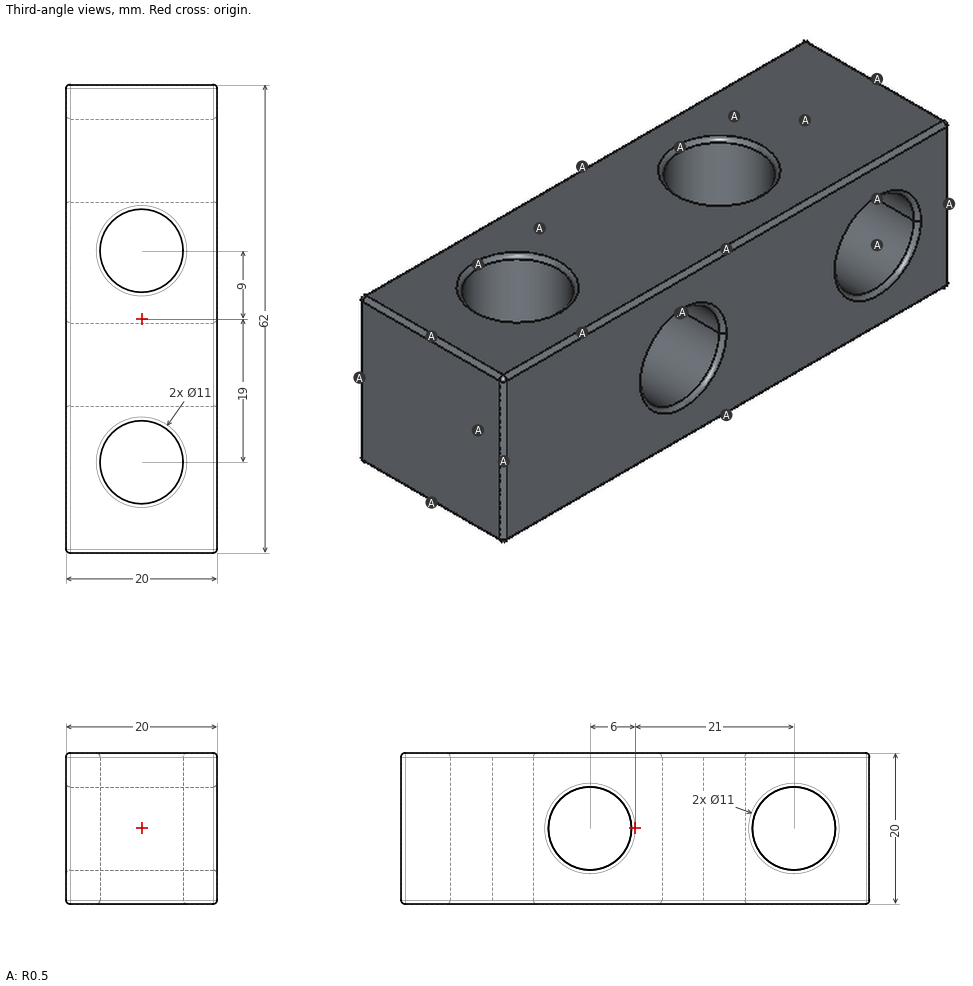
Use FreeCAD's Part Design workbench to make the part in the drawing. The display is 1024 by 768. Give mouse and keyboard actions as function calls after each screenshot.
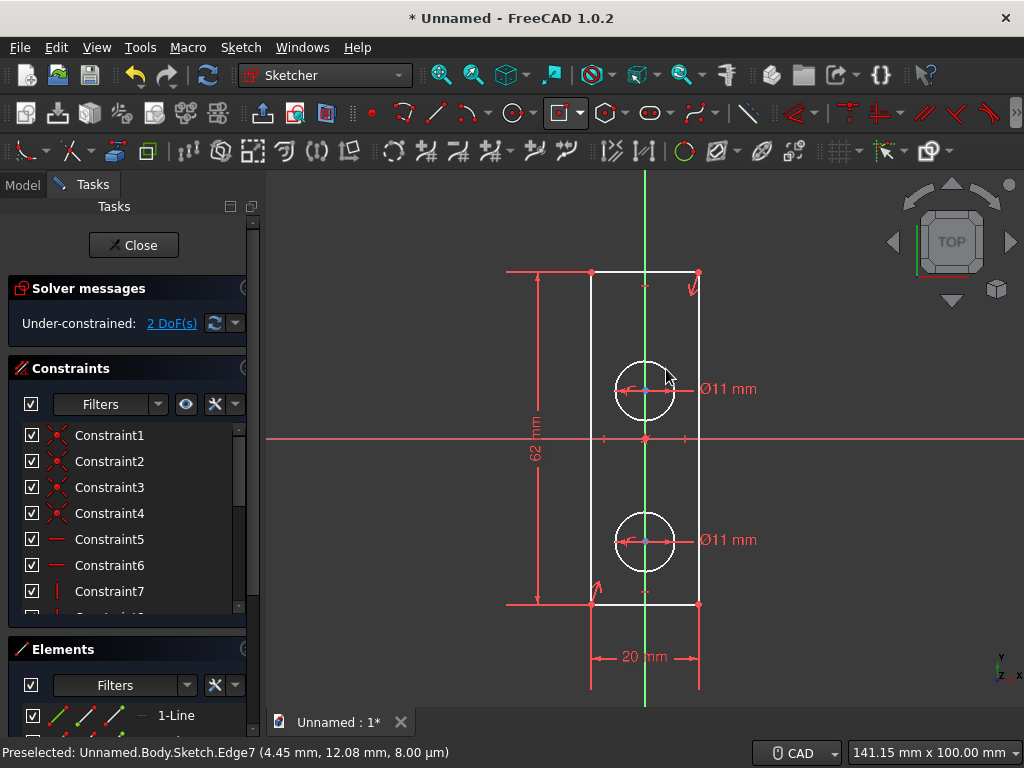
key(d)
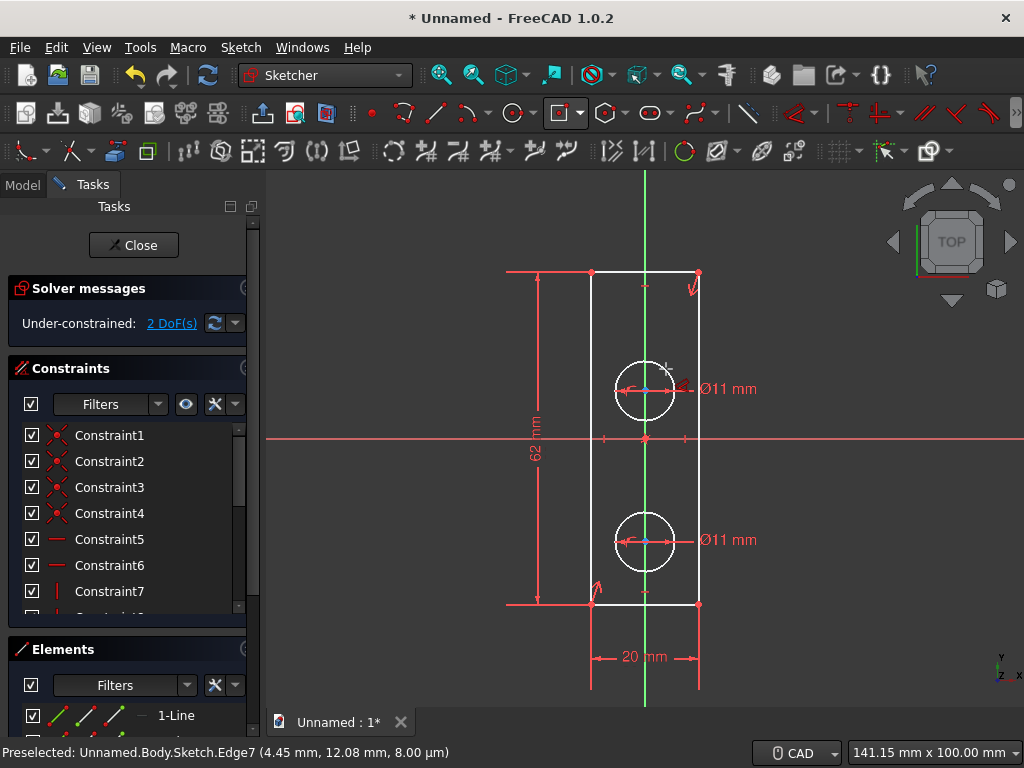
click(645, 391)
click(727, 415)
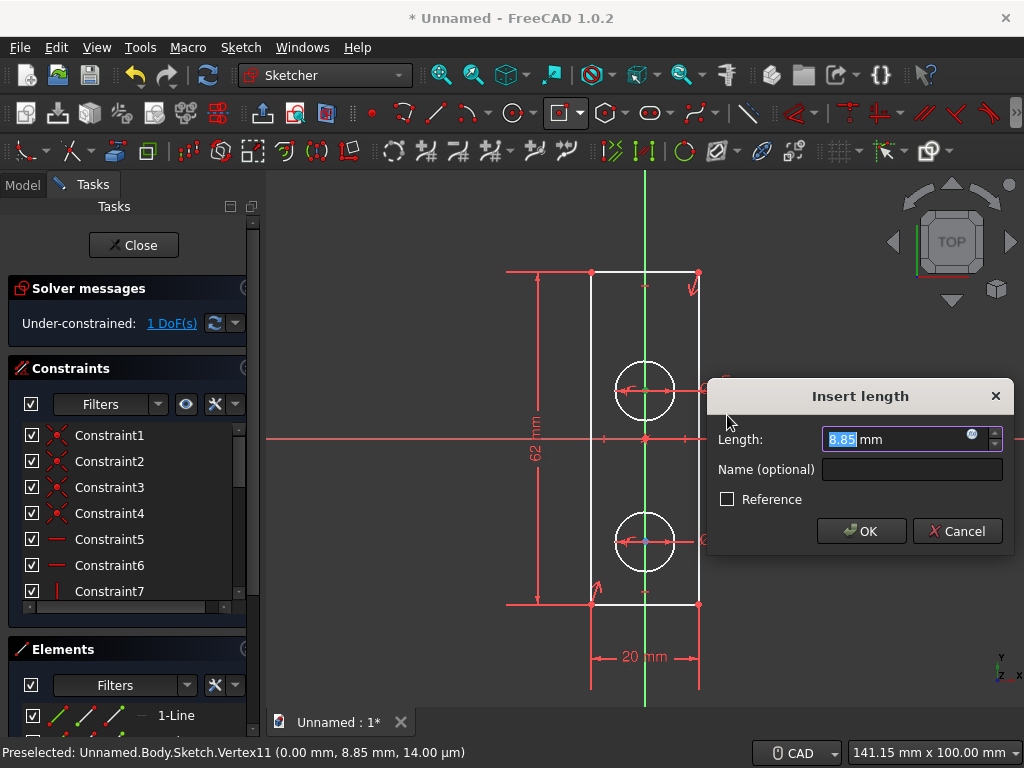
text(9)
key(Return)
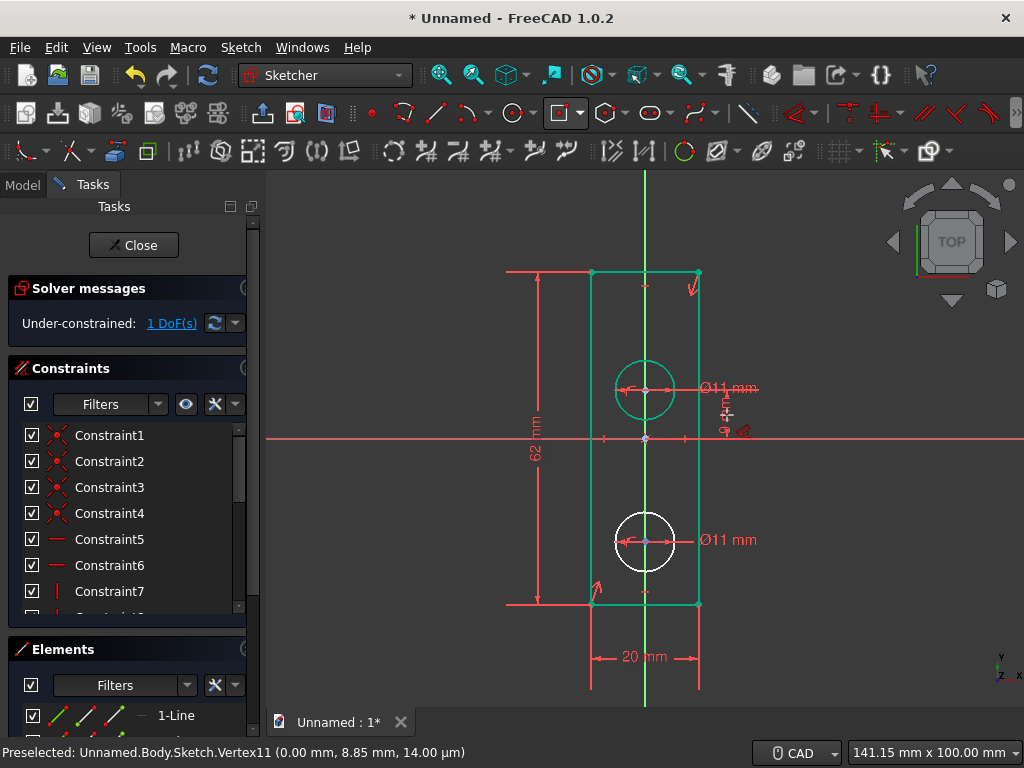
click(645, 542)
click(679, 490)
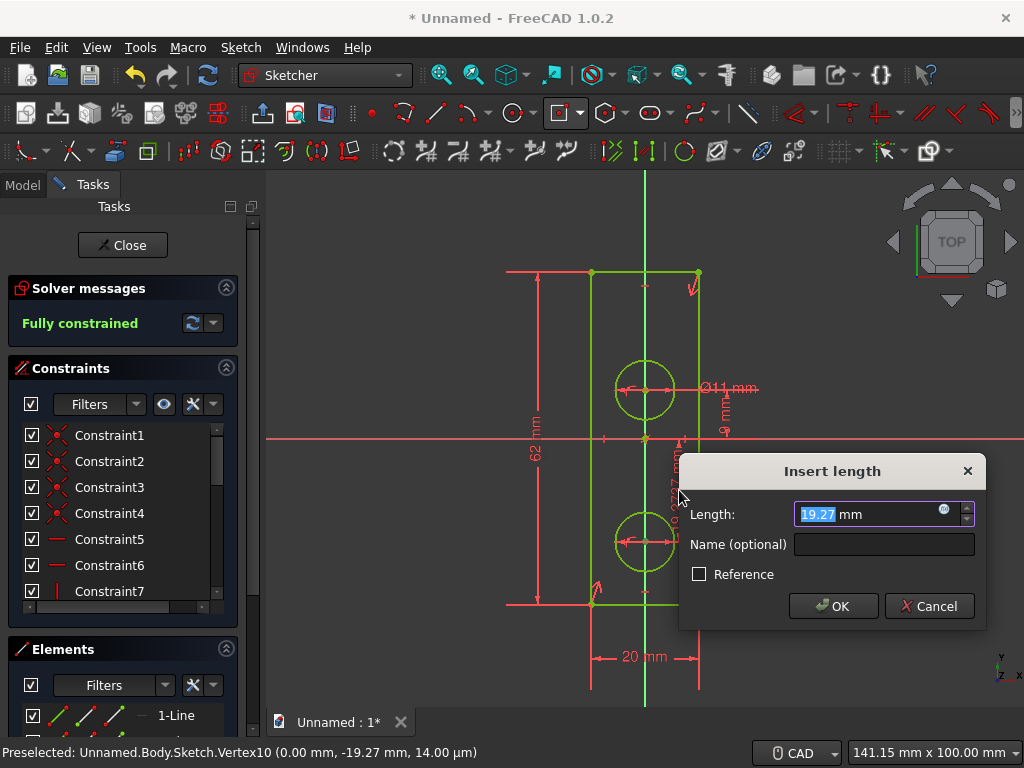
text(19)
key(Return)
key(Escape)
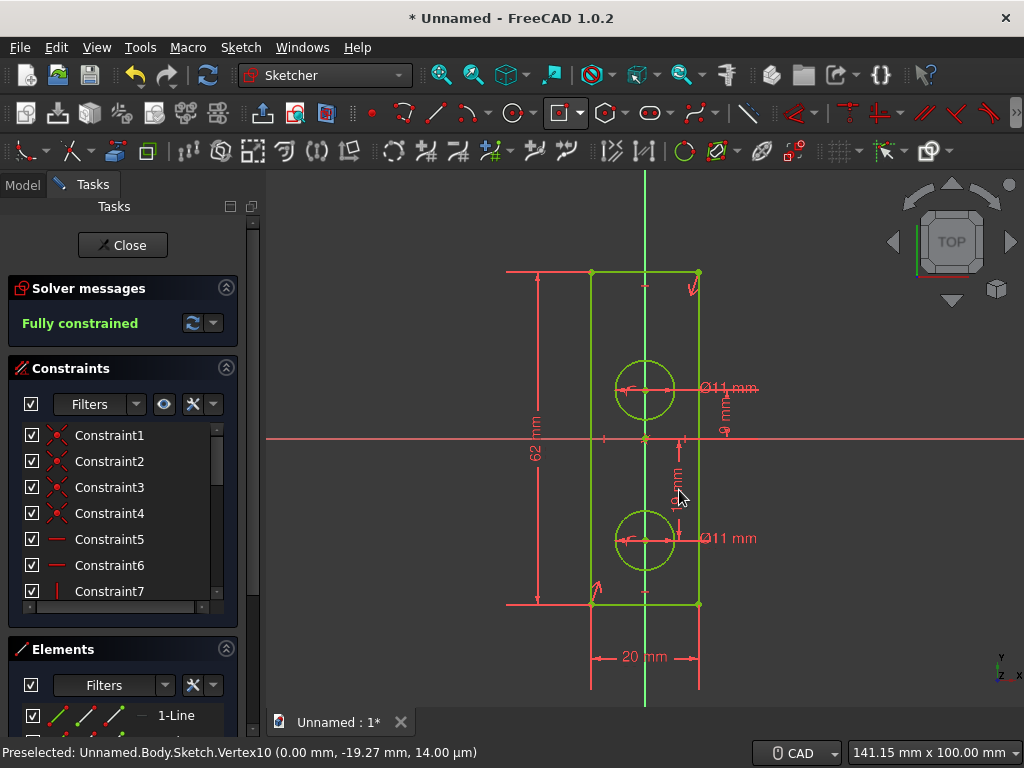
click(123, 245)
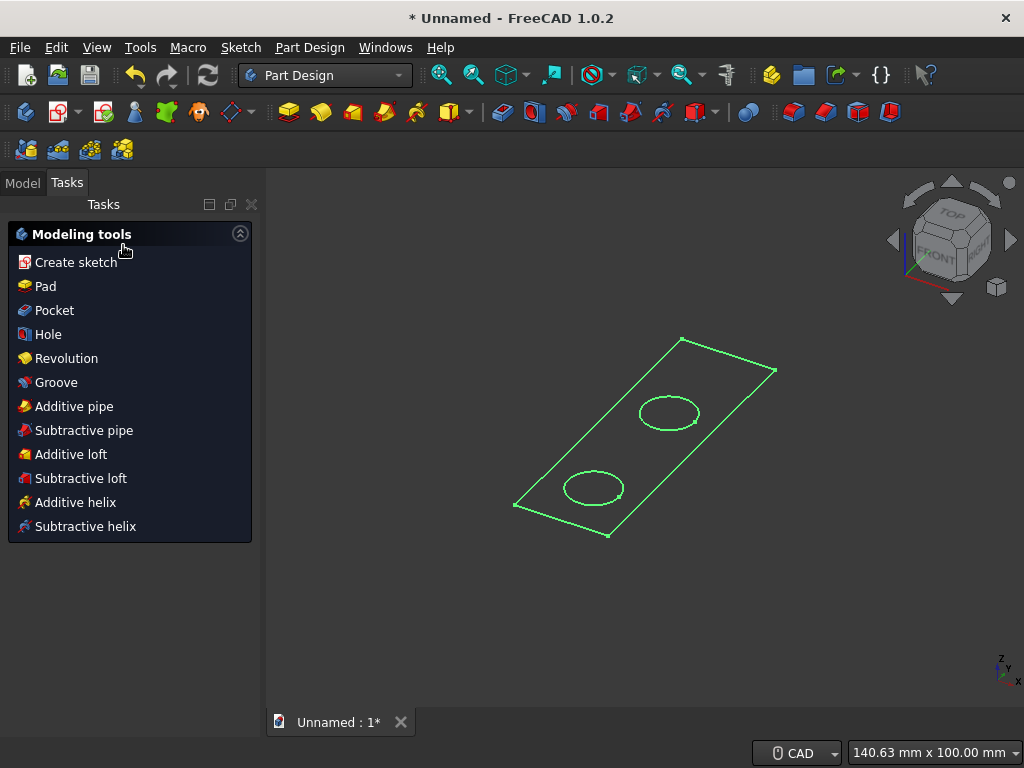
click(290, 112)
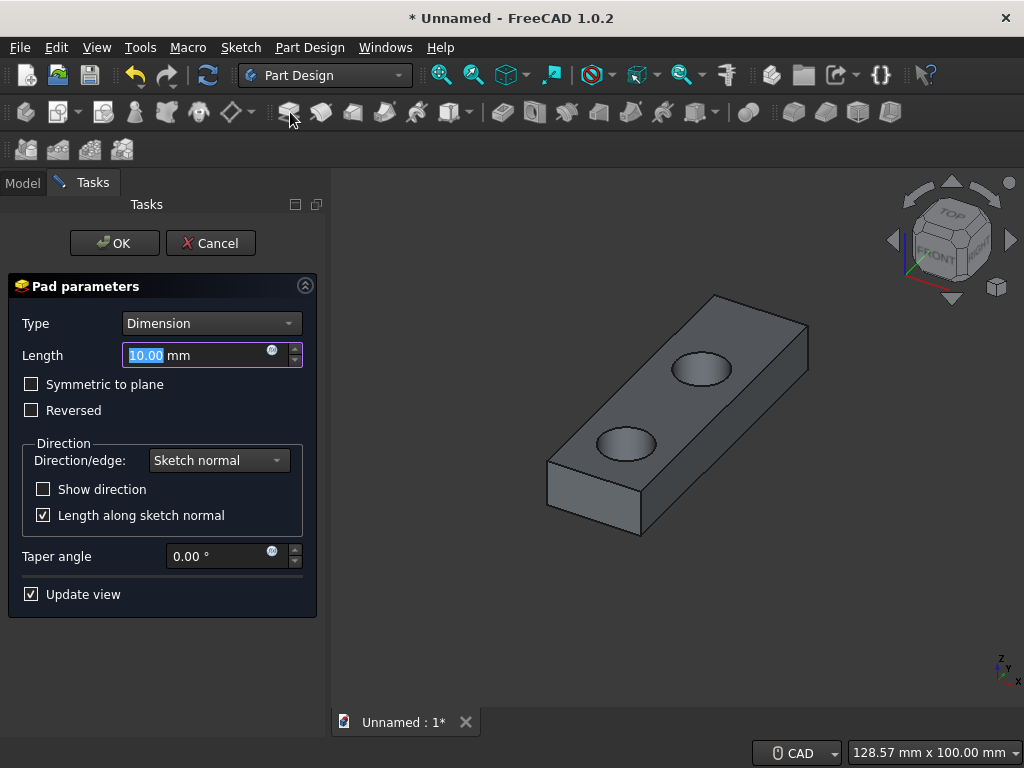
text(20)
key(Tab)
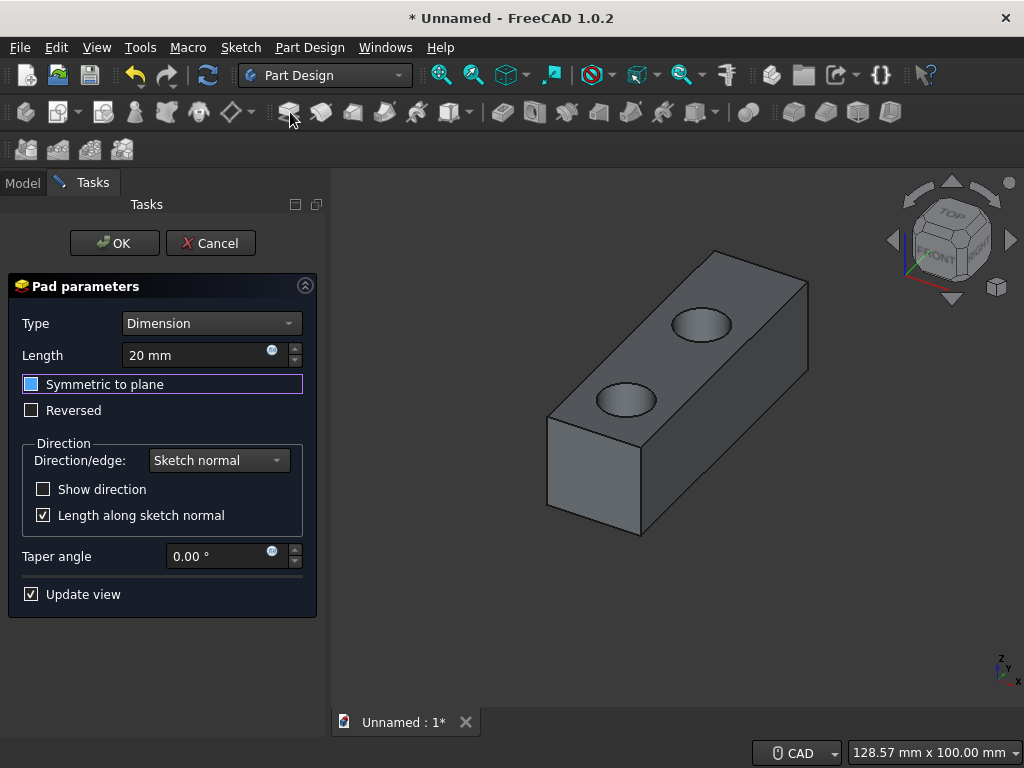
click(30, 384)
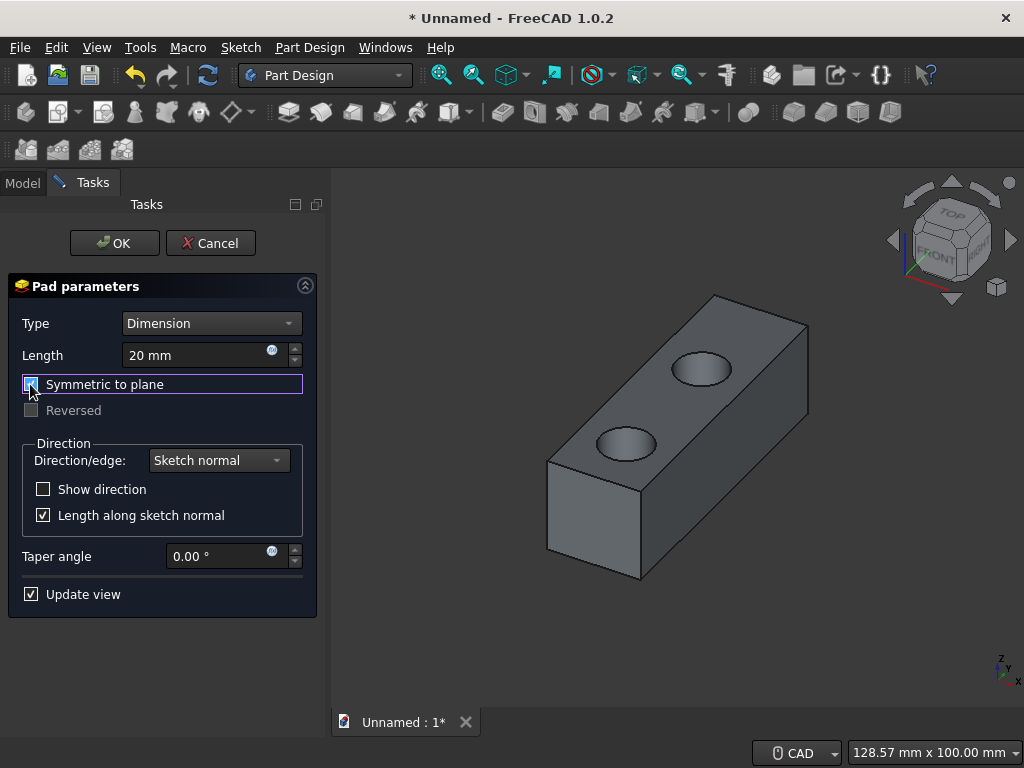
click(115, 243)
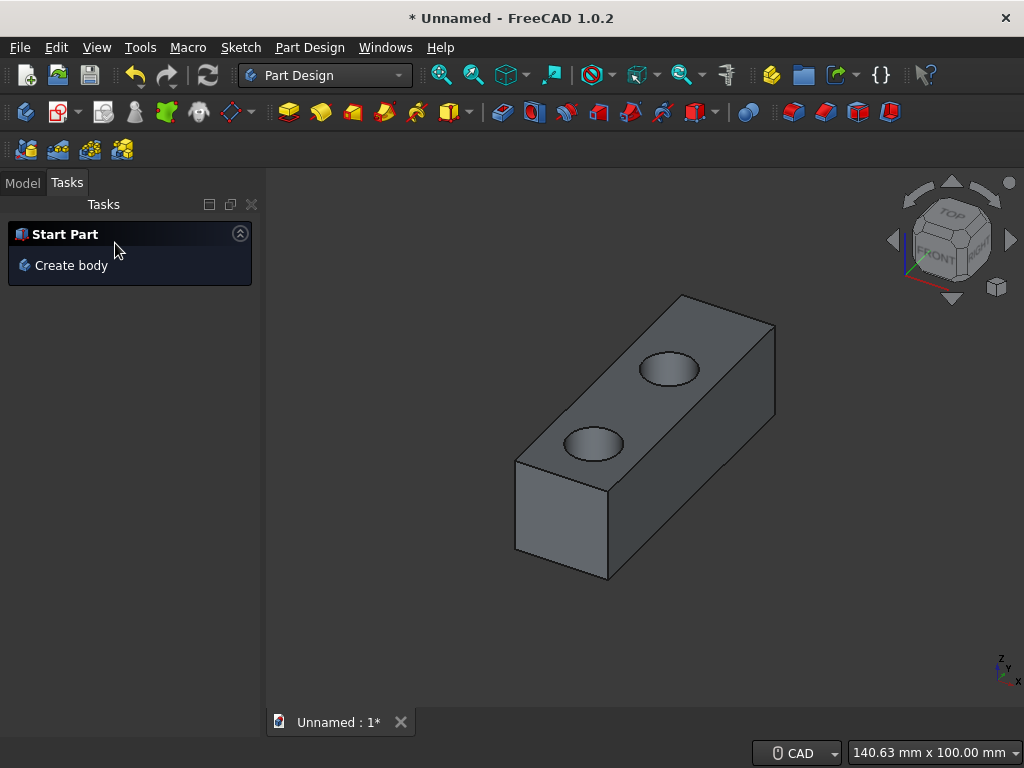
click(739, 405)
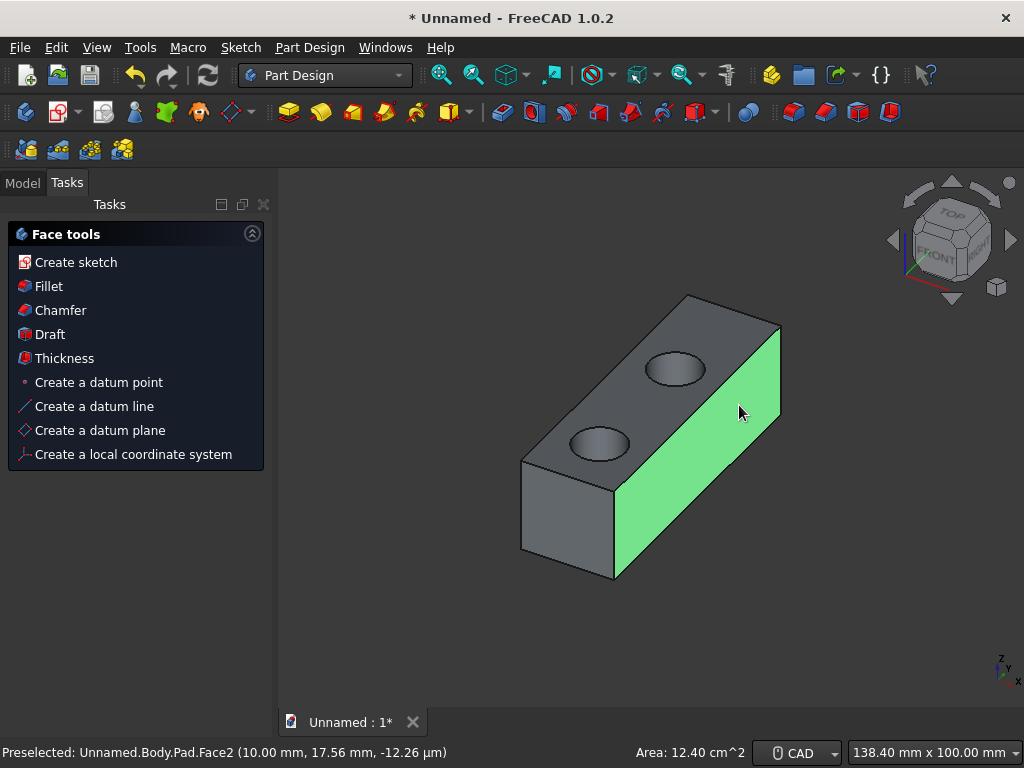
click(58, 112)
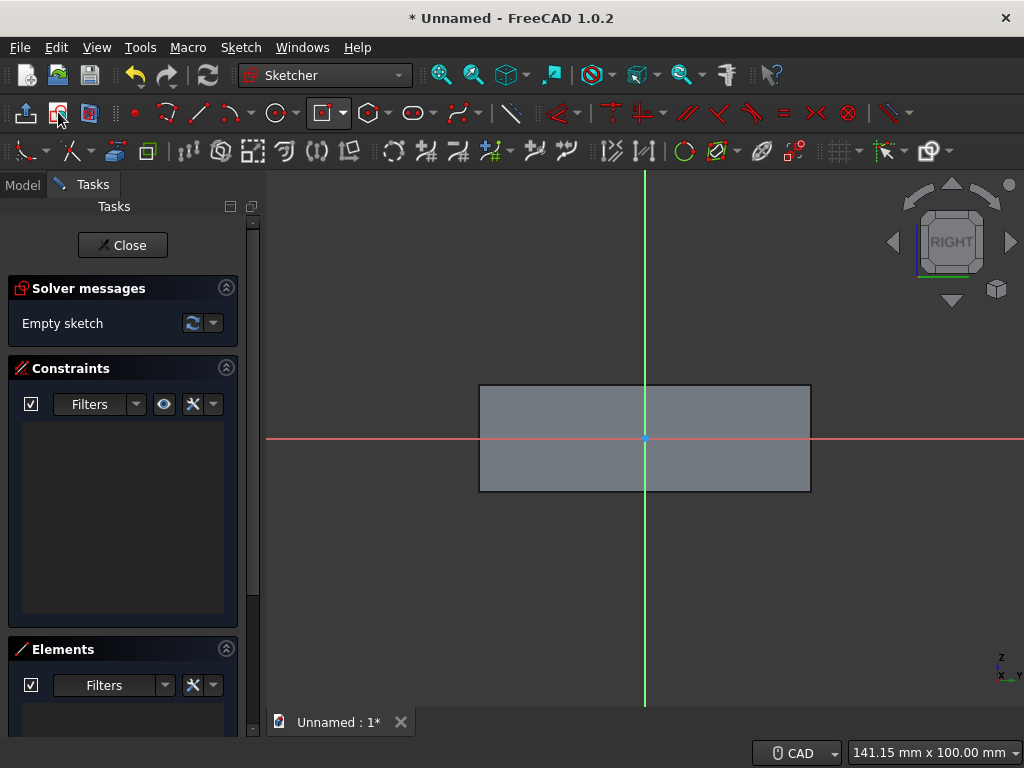
scroll(818, 438, up, 3)